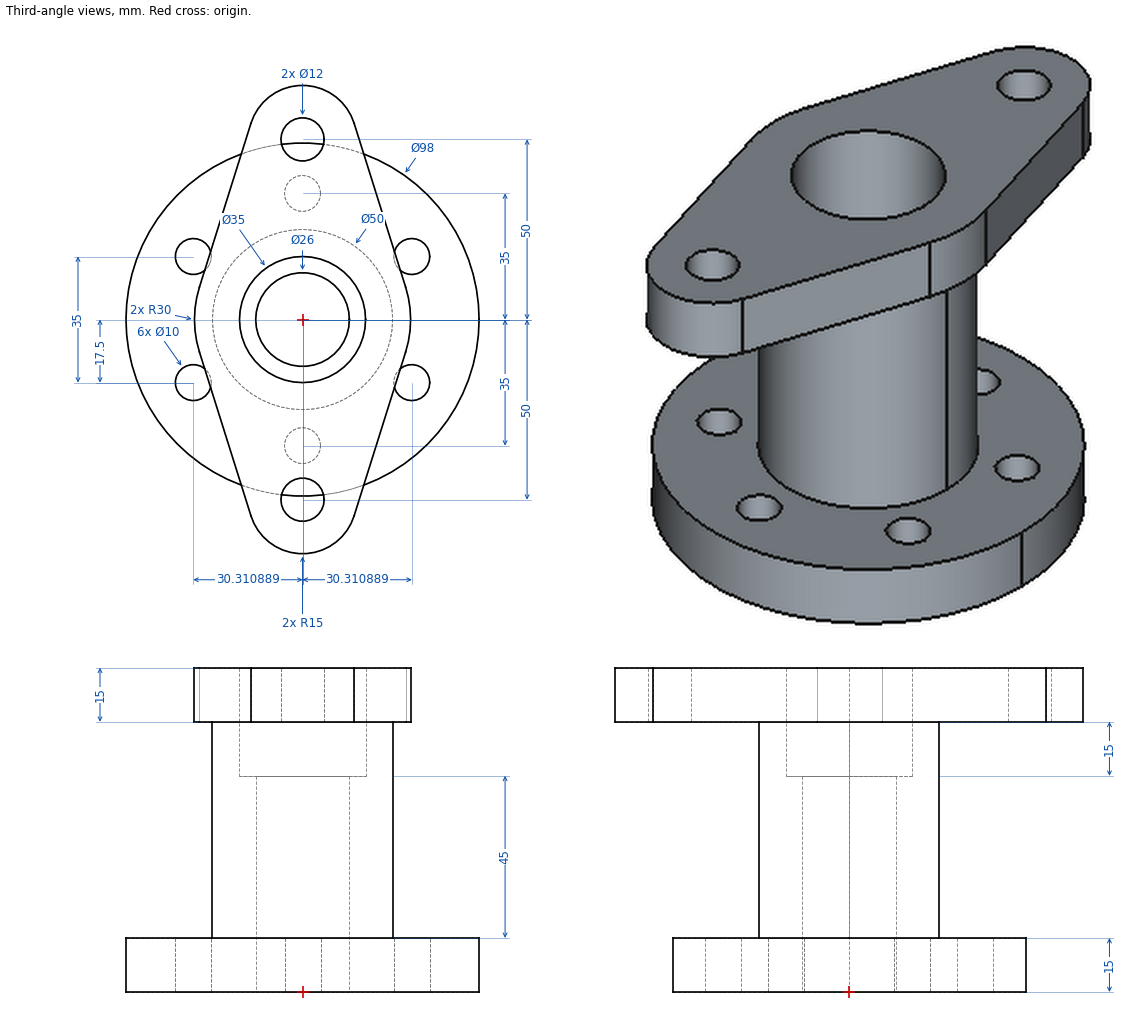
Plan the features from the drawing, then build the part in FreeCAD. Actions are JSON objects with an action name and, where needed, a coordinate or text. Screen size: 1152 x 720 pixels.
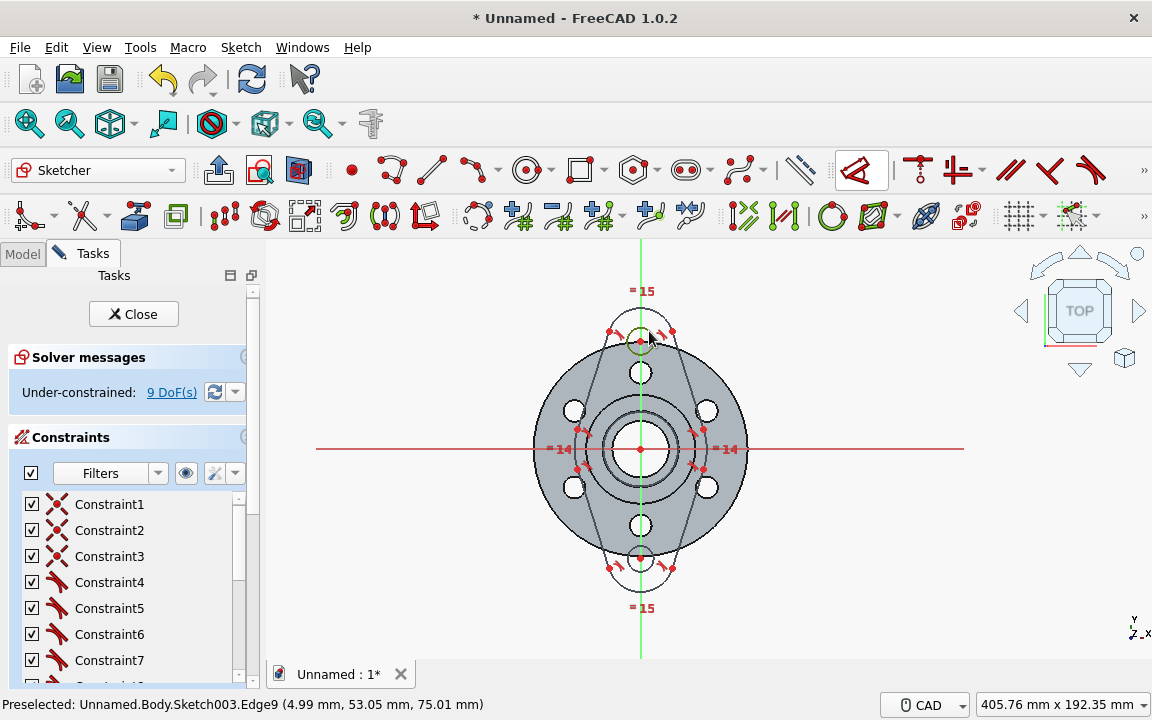
{"action": "scroll", "coordinate": [650, 550], "scroll_direction": "up", "scroll_amount": 3}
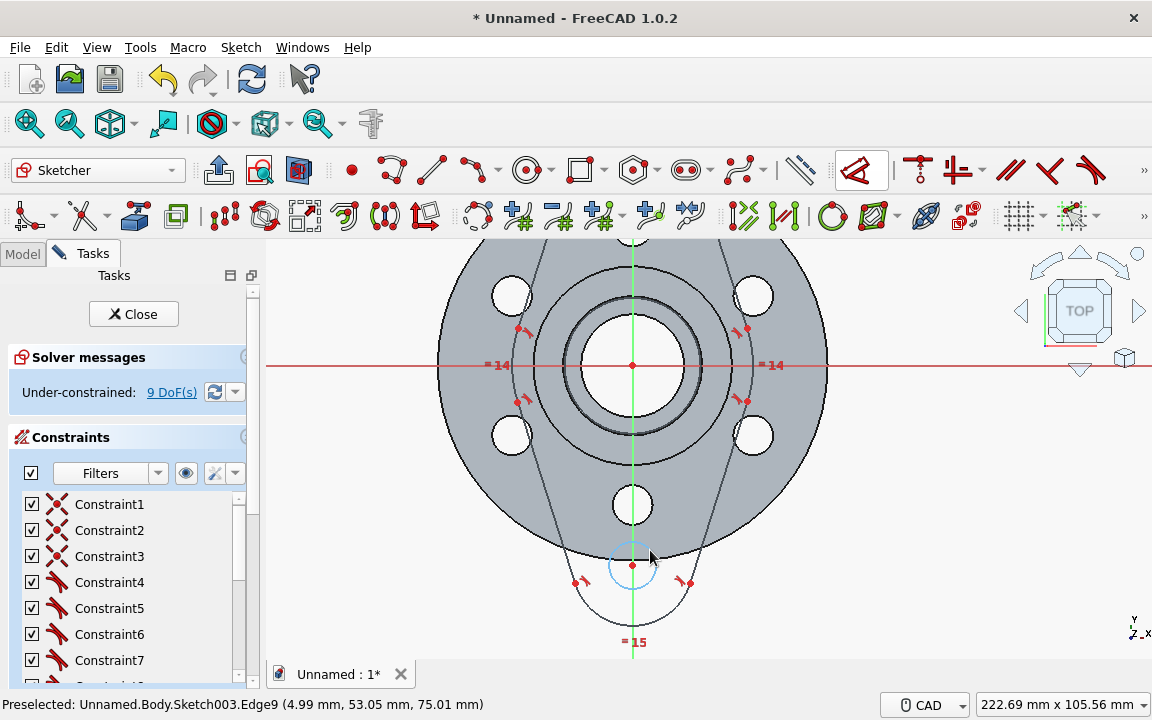
{"action": "left_click", "coordinate": [649, 549]}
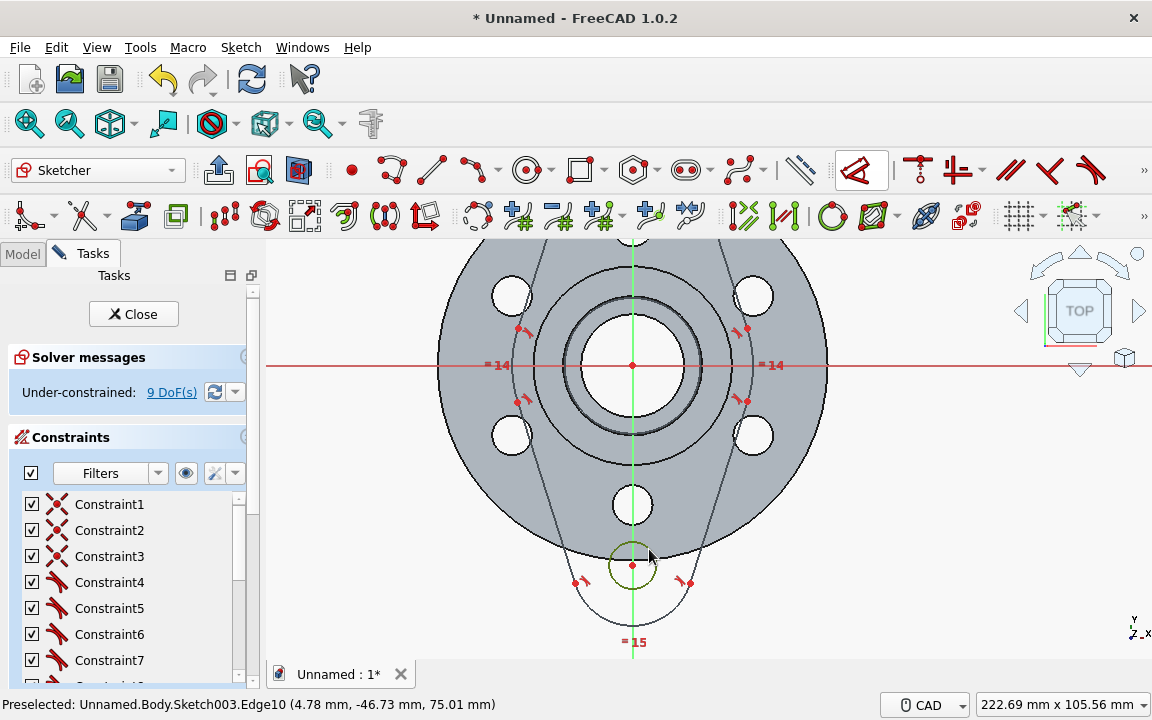
{"action": "key", "text": "e"}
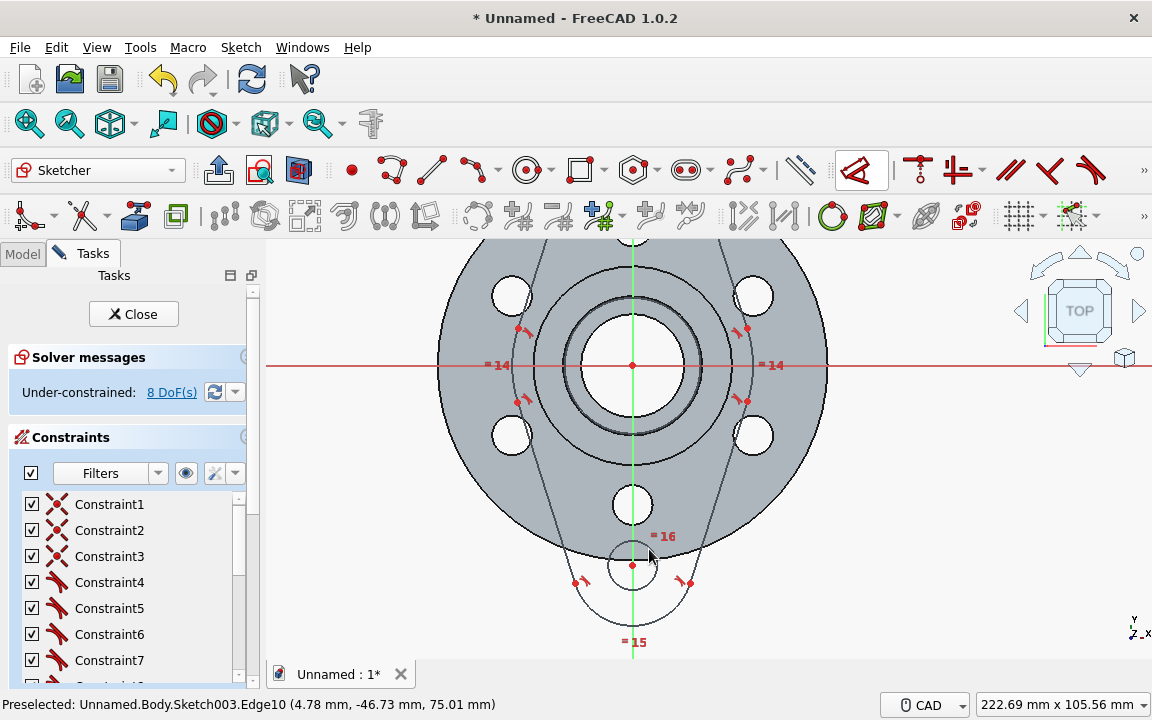
{"action": "left_click", "coordinate": [633, 566]}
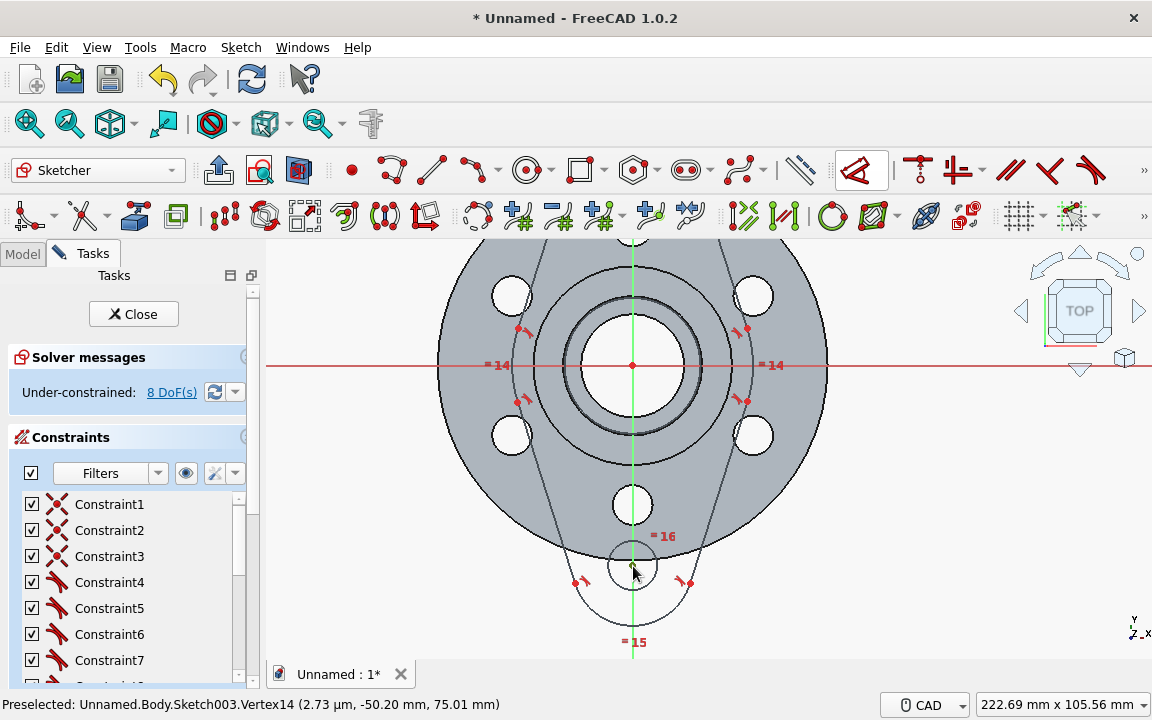
{"action": "left_click", "coordinate": [633, 501]}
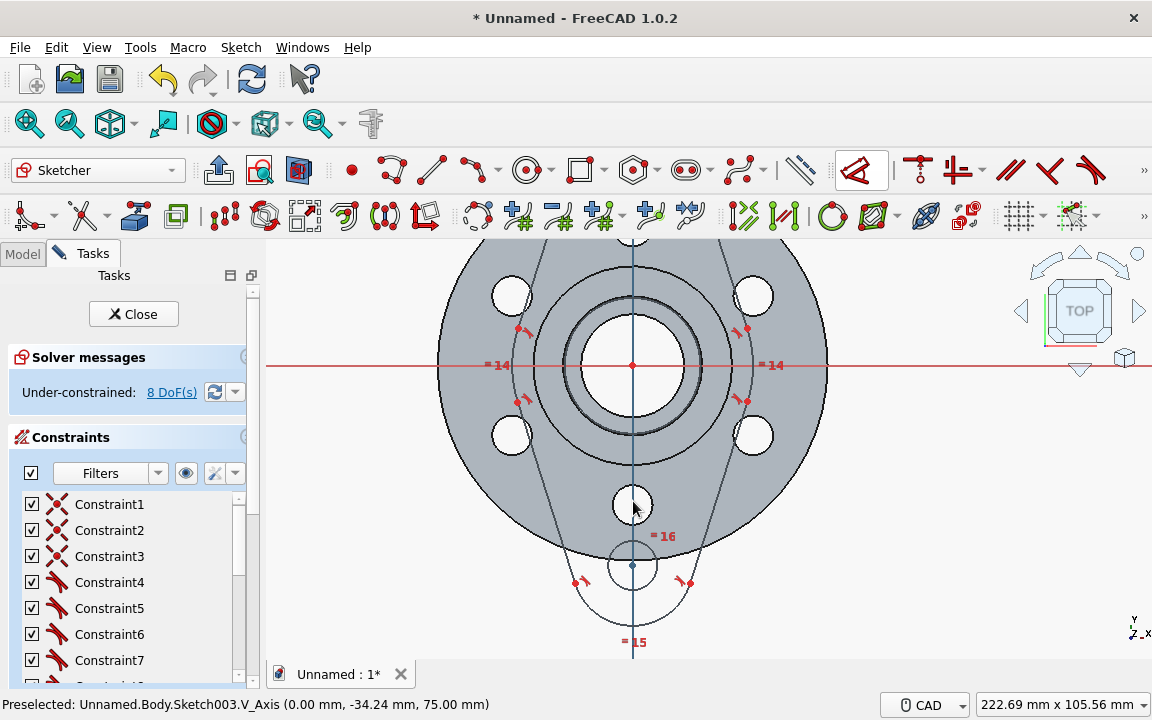
{"action": "left_click", "coordinate": [918, 170]}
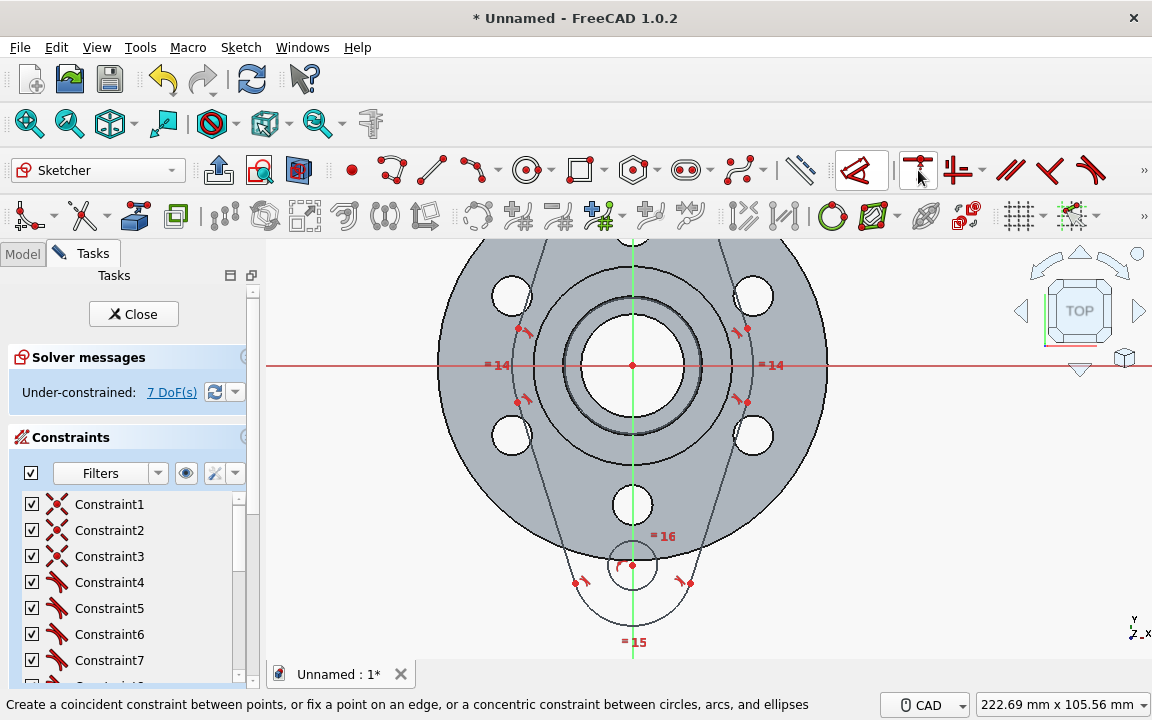
{"action": "scroll", "coordinate": [650, 550], "scroll_direction": "down", "scroll_amount": 3}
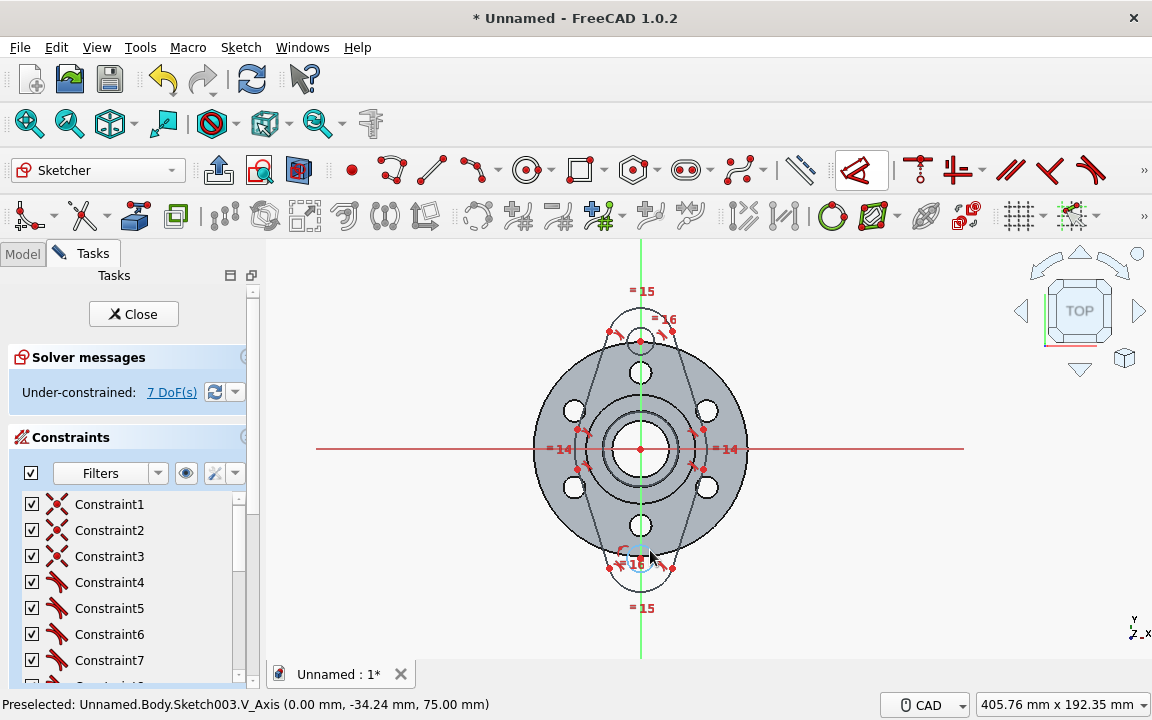
{"action": "left_click", "coordinate": [641, 341]}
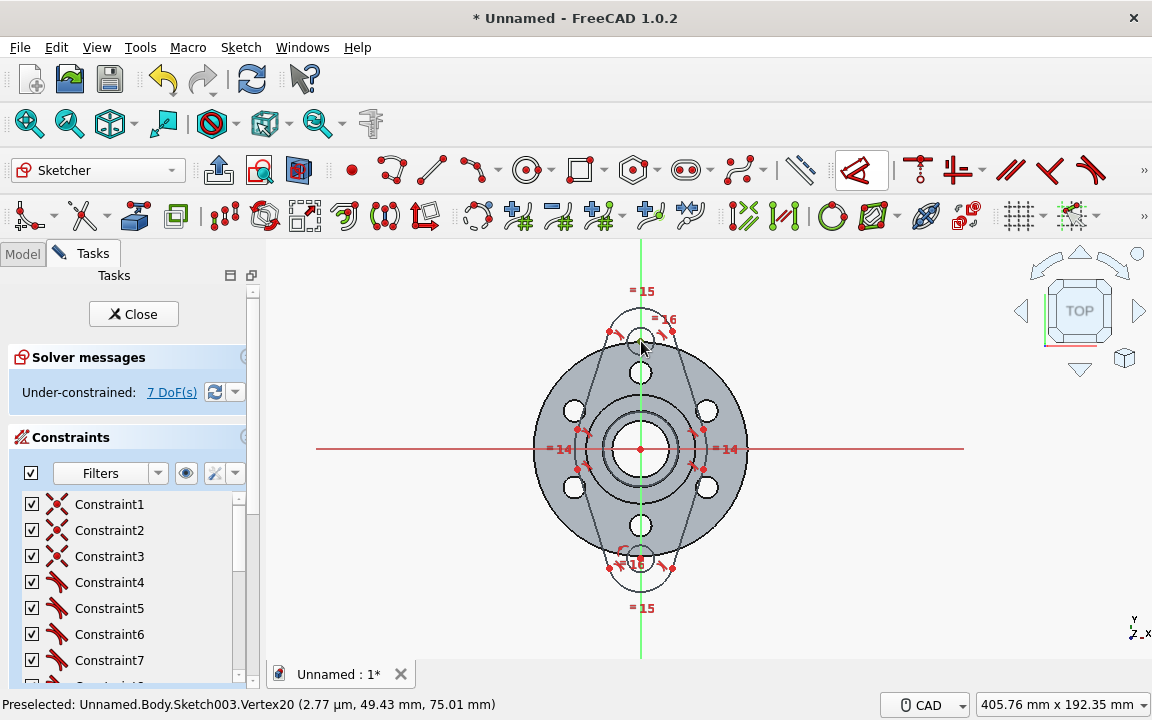
{"action": "left_click", "coordinate": [641, 527]}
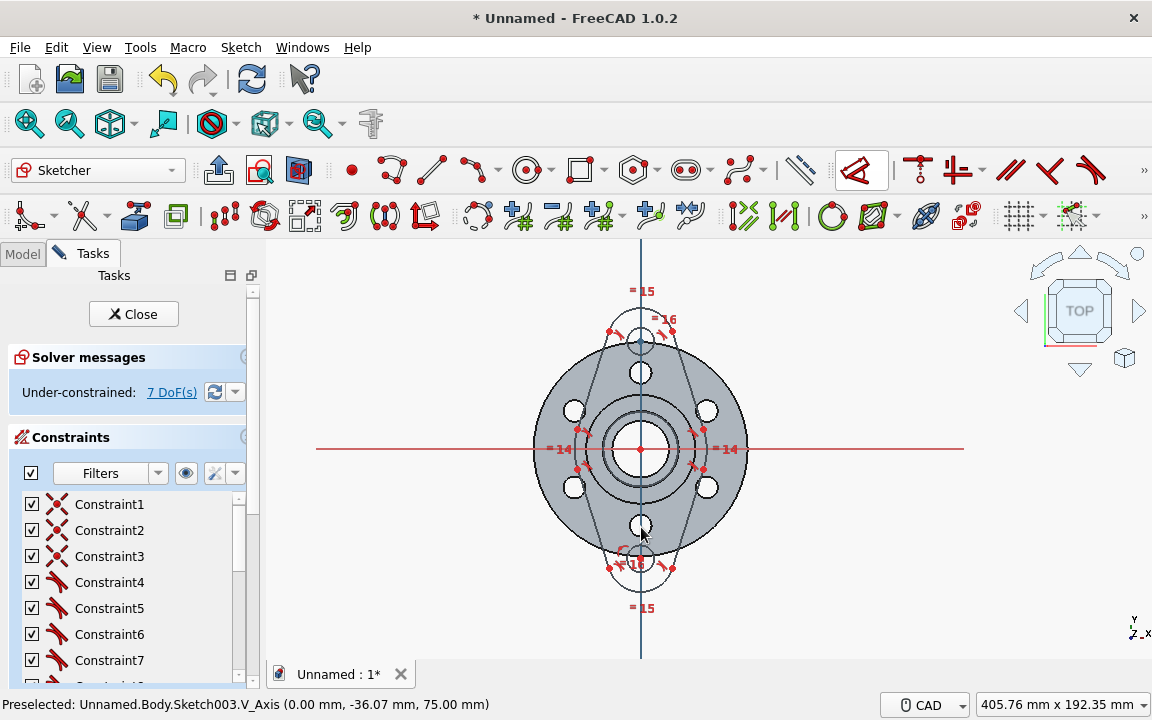
{"action": "key", "text": "c"}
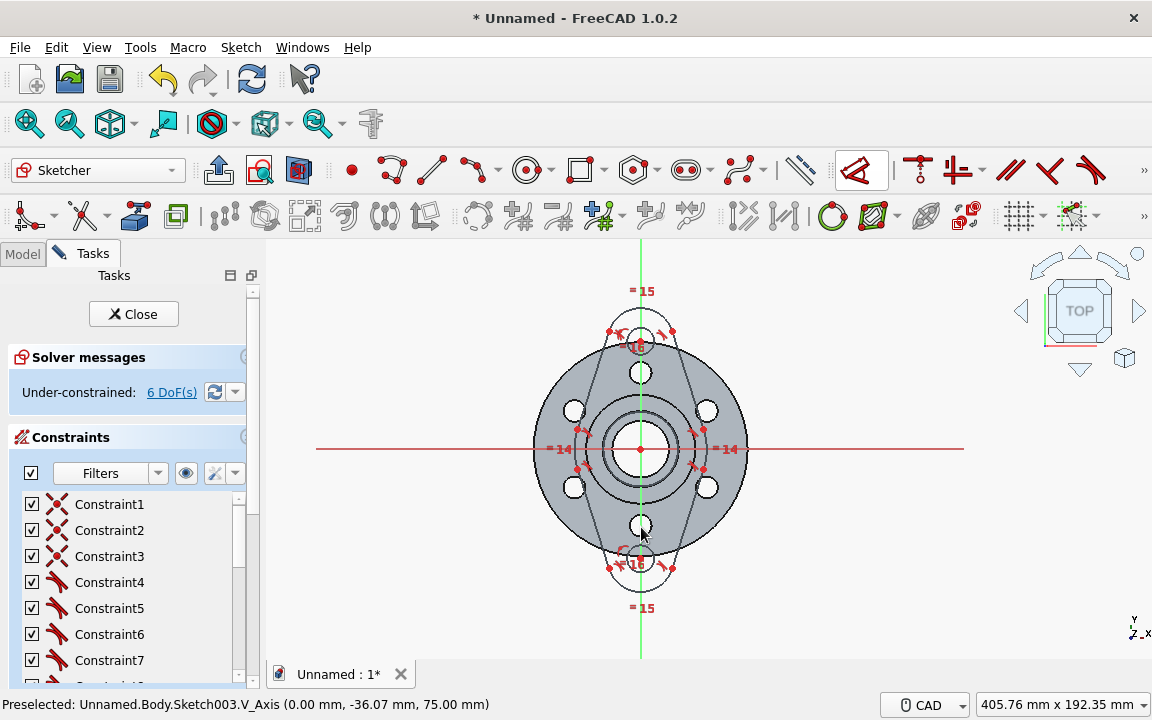
{"action": "left_click", "coordinate": [575, 449]}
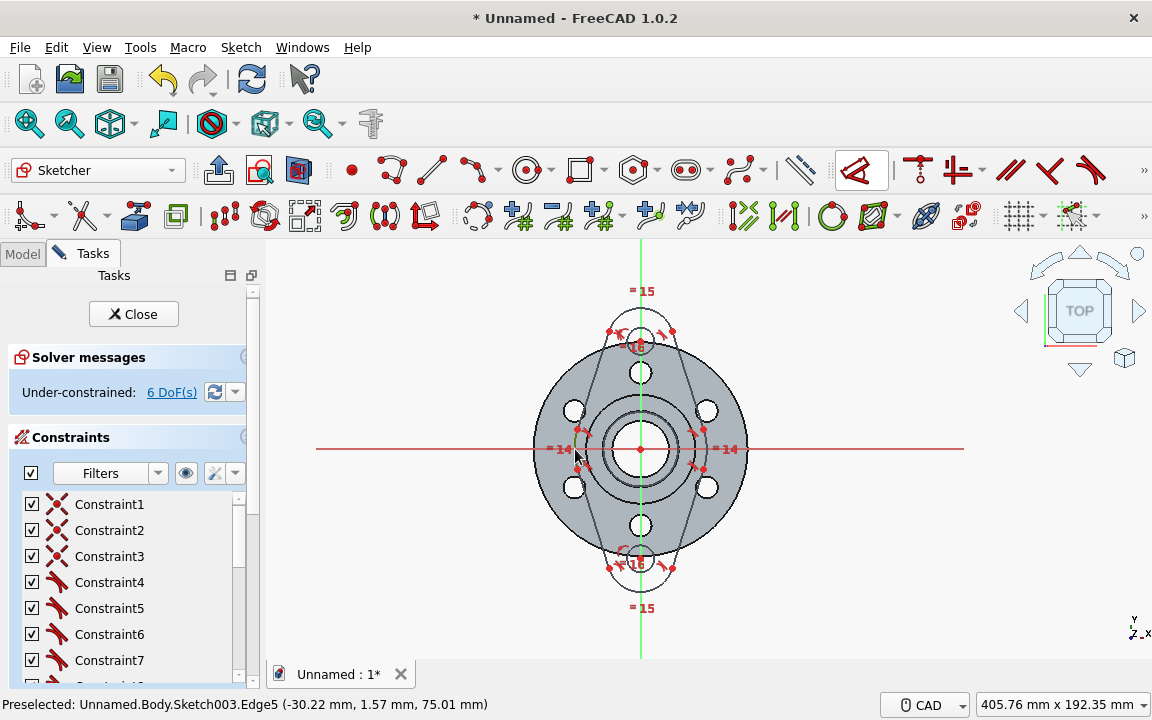
{"action": "key", "text": "k r"}